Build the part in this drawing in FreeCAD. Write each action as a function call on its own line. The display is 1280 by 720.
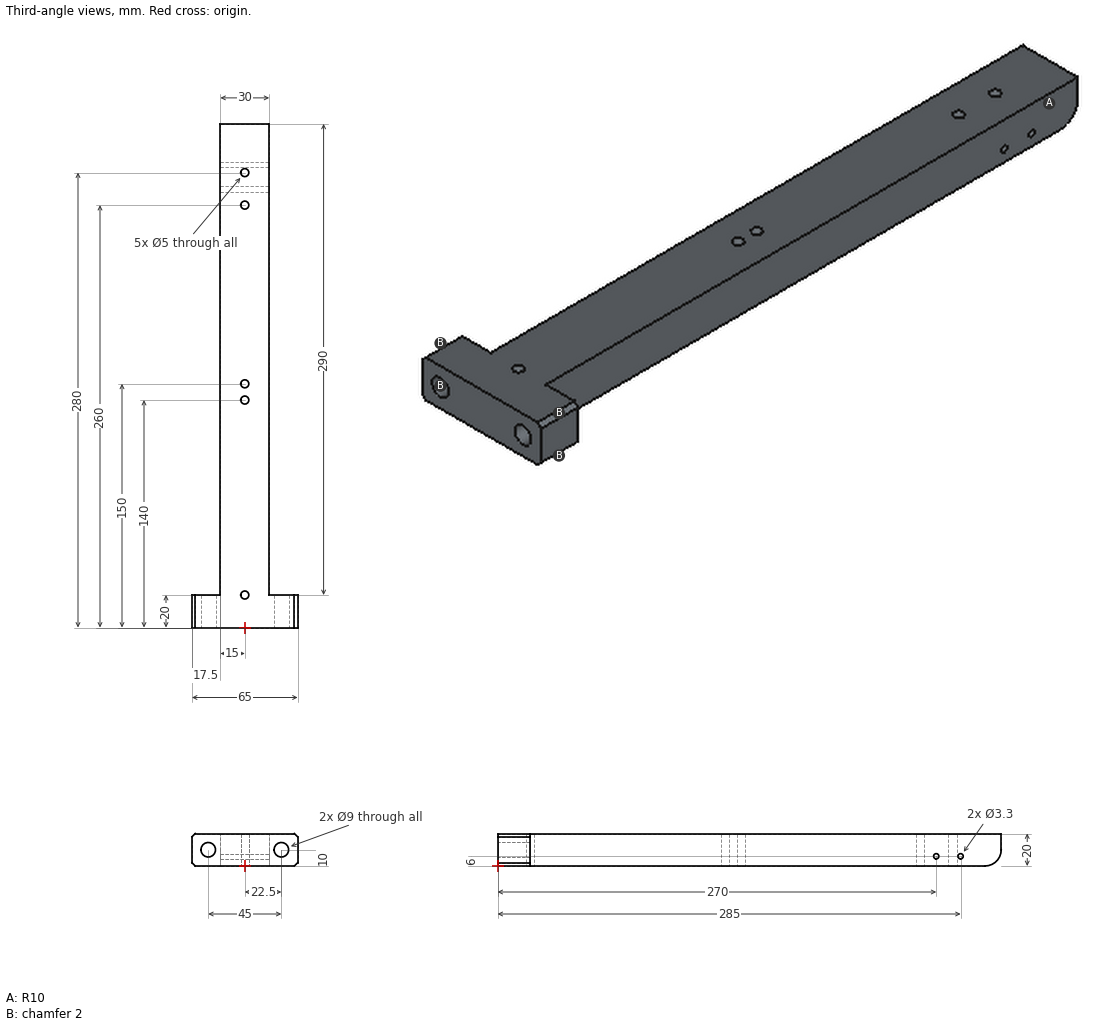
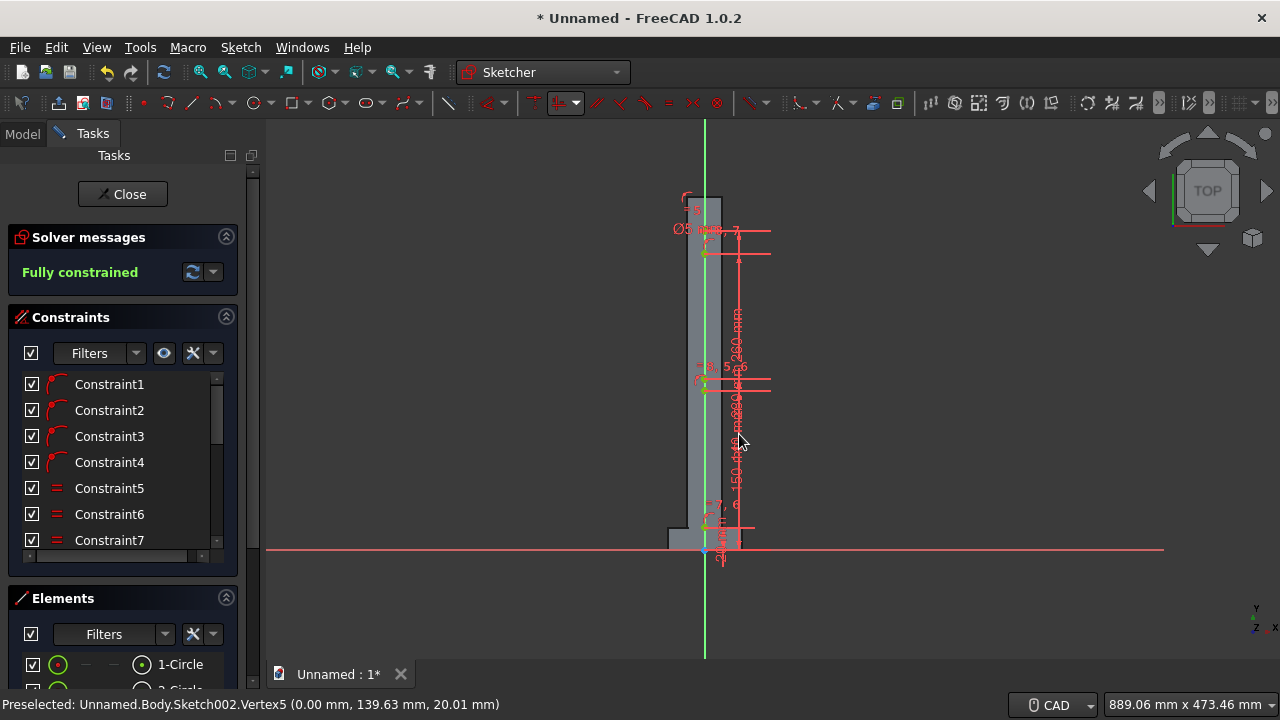
click(123, 194)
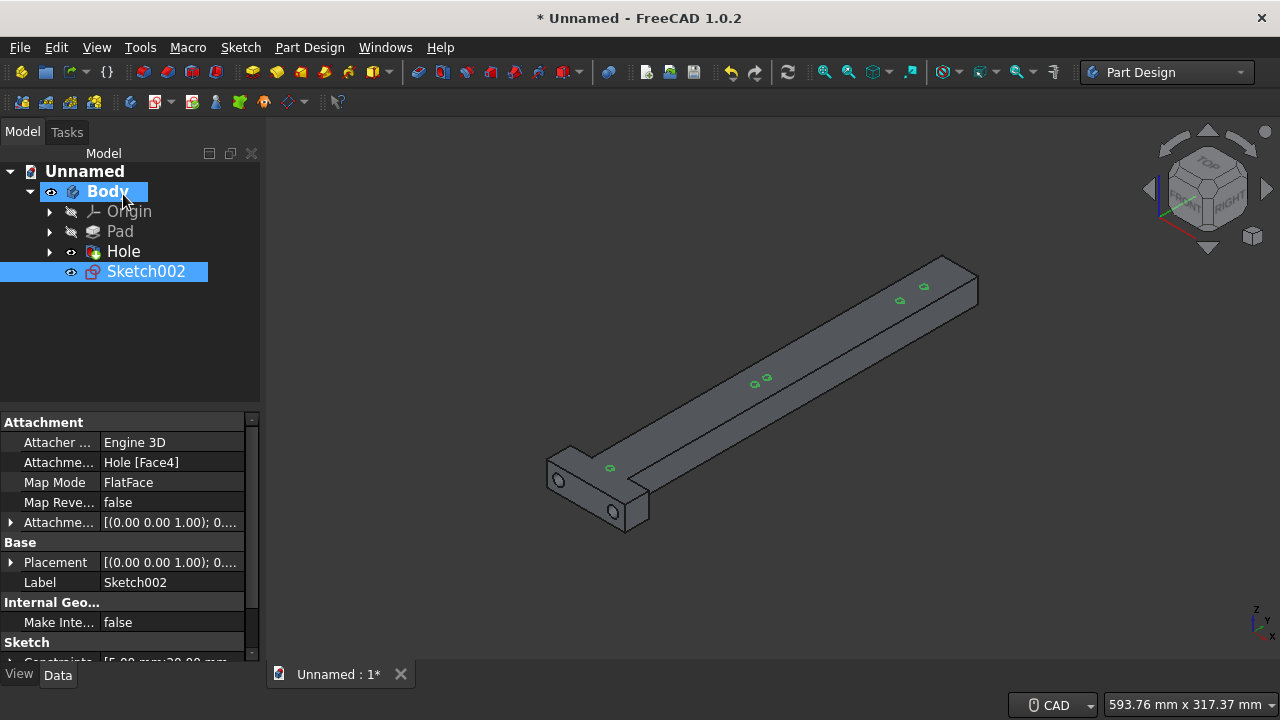
click(444, 72)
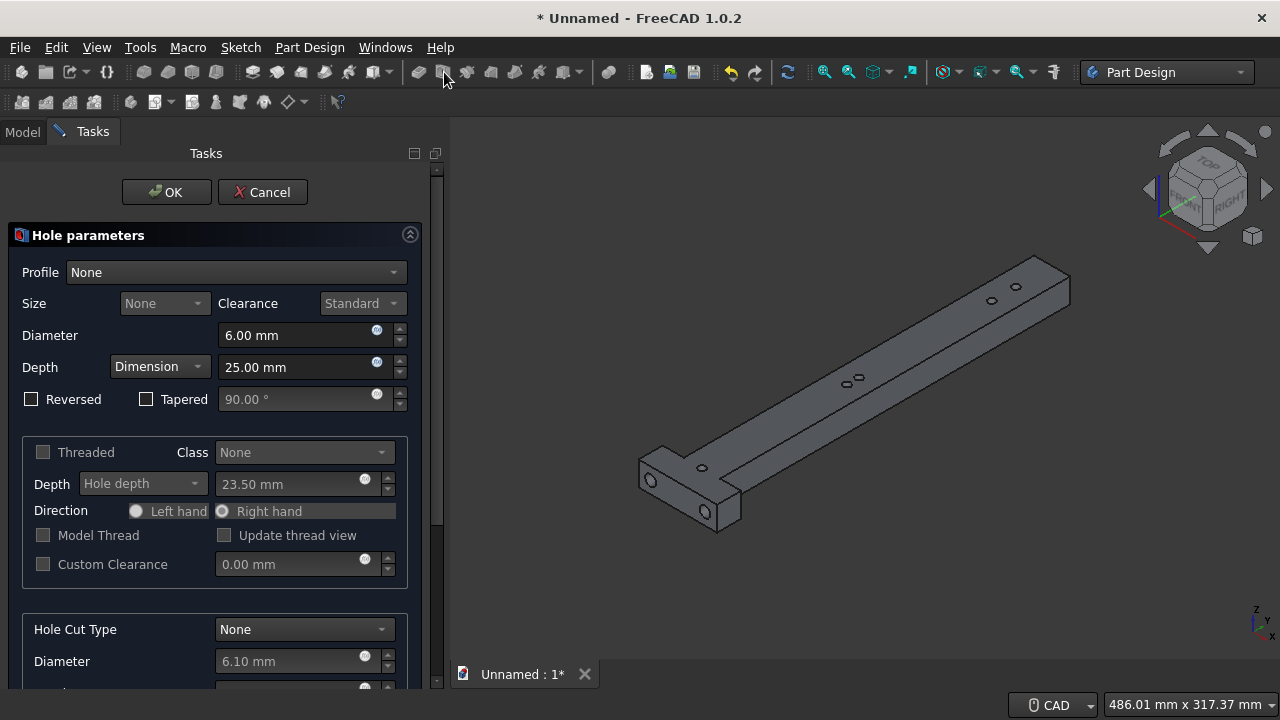
triple_click(305, 335)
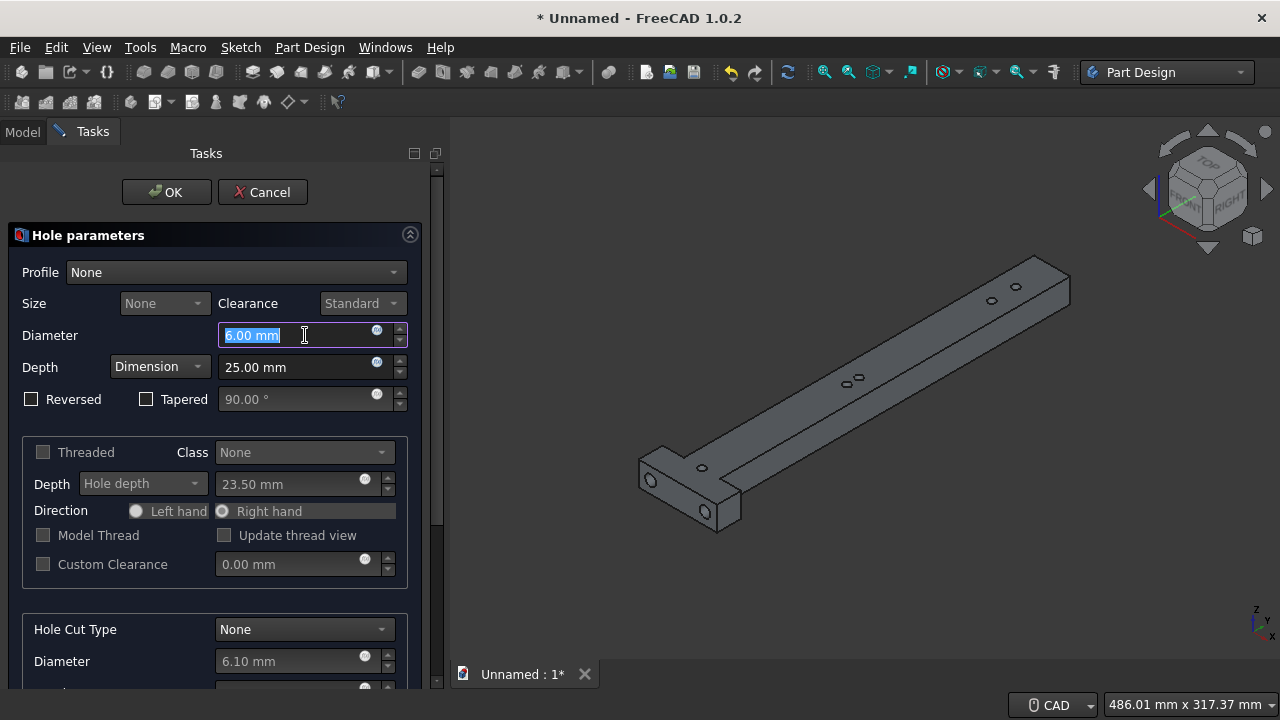
text(5)
key(Tab)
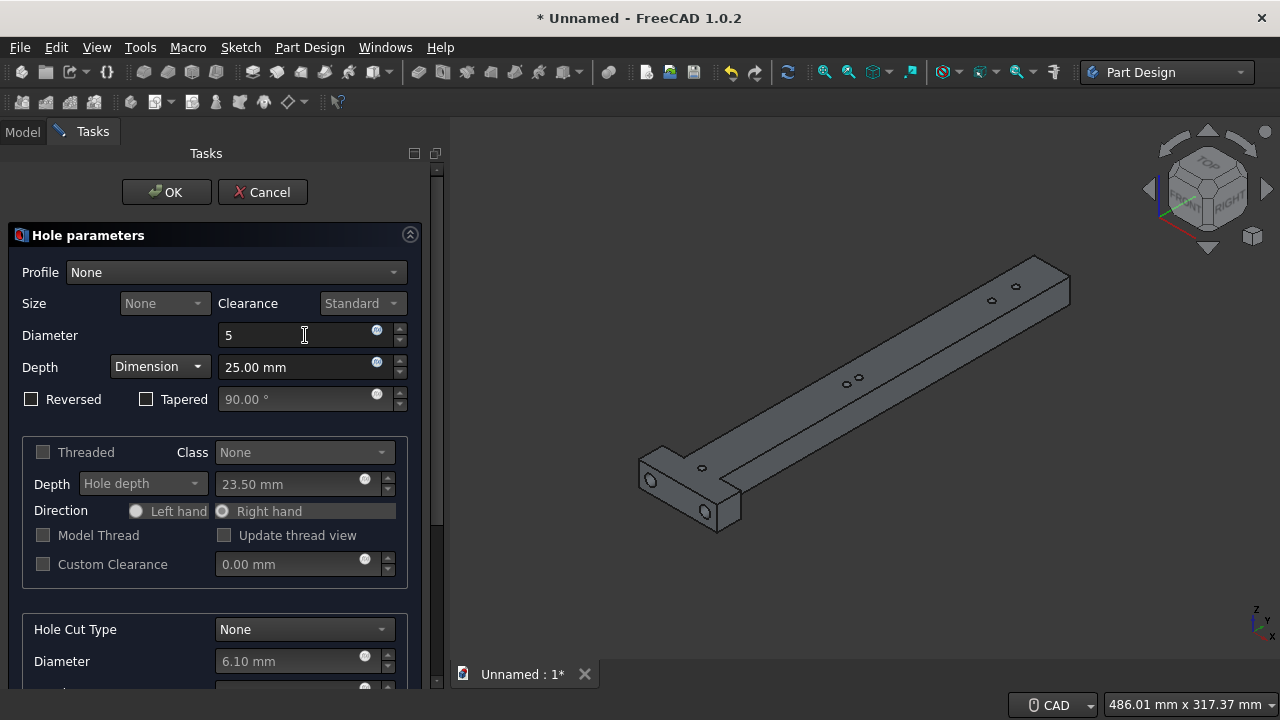
click(161, 366)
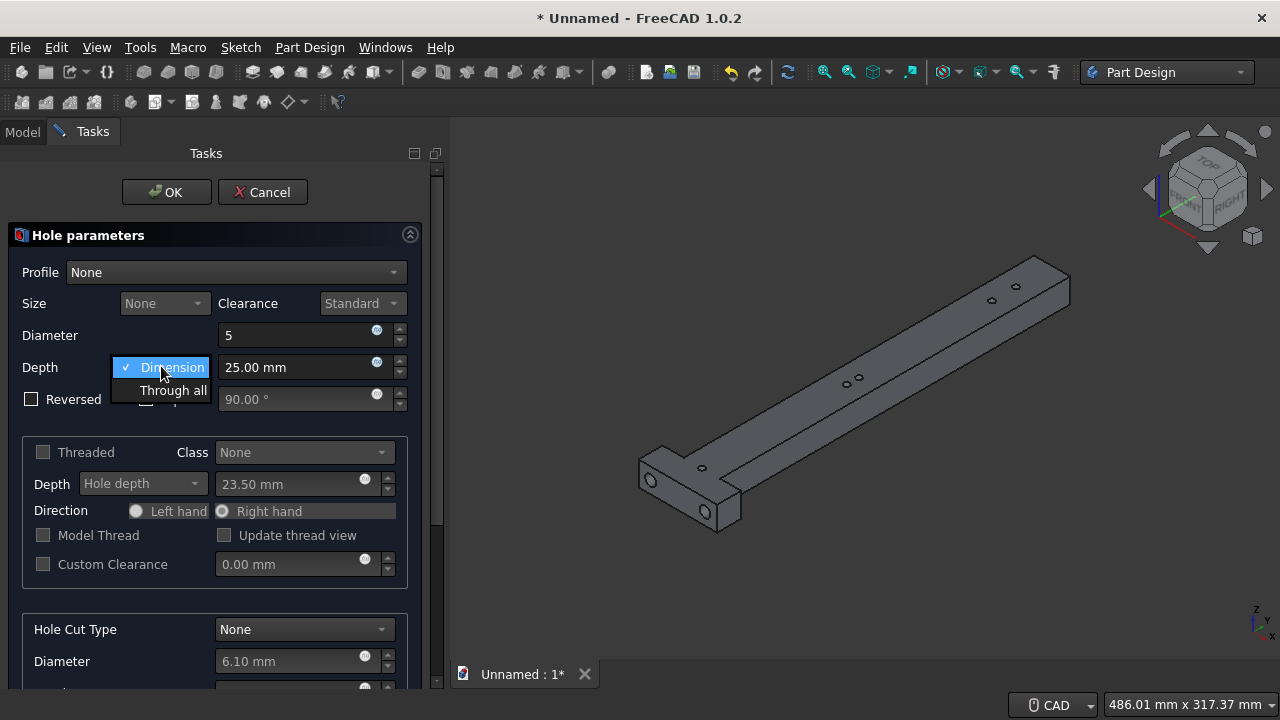
click(160, 390)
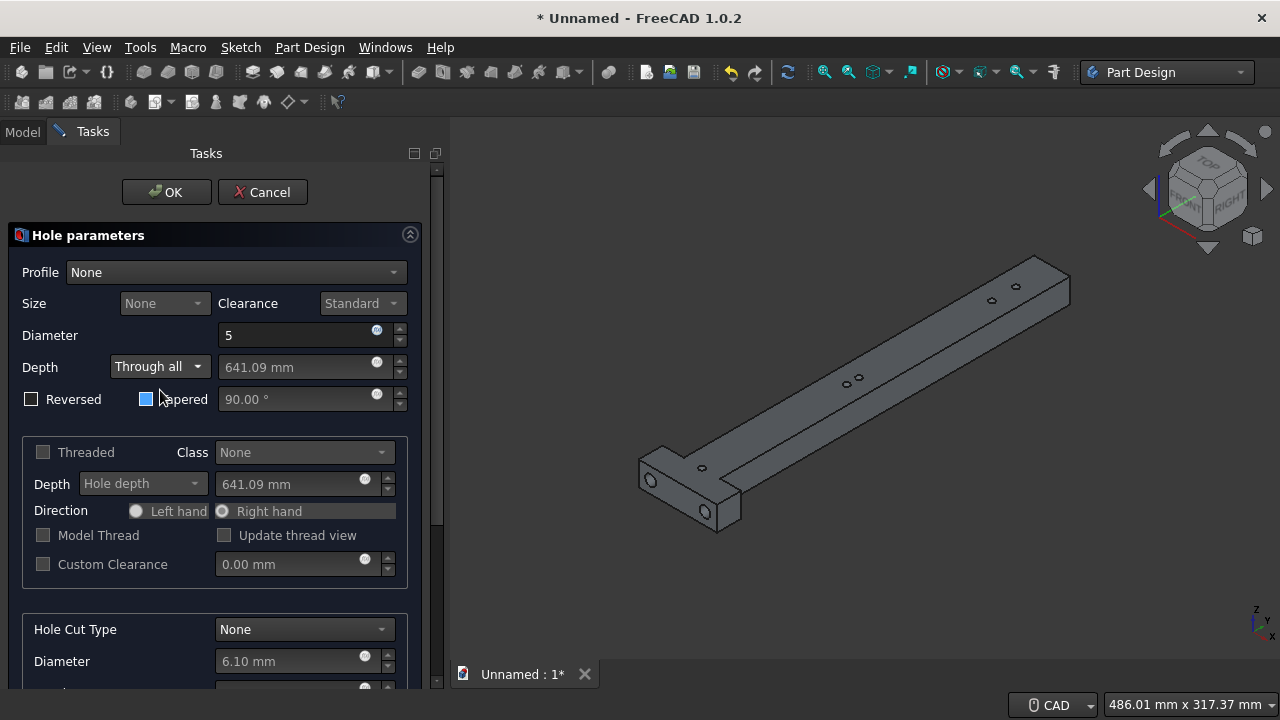
click(167, 192)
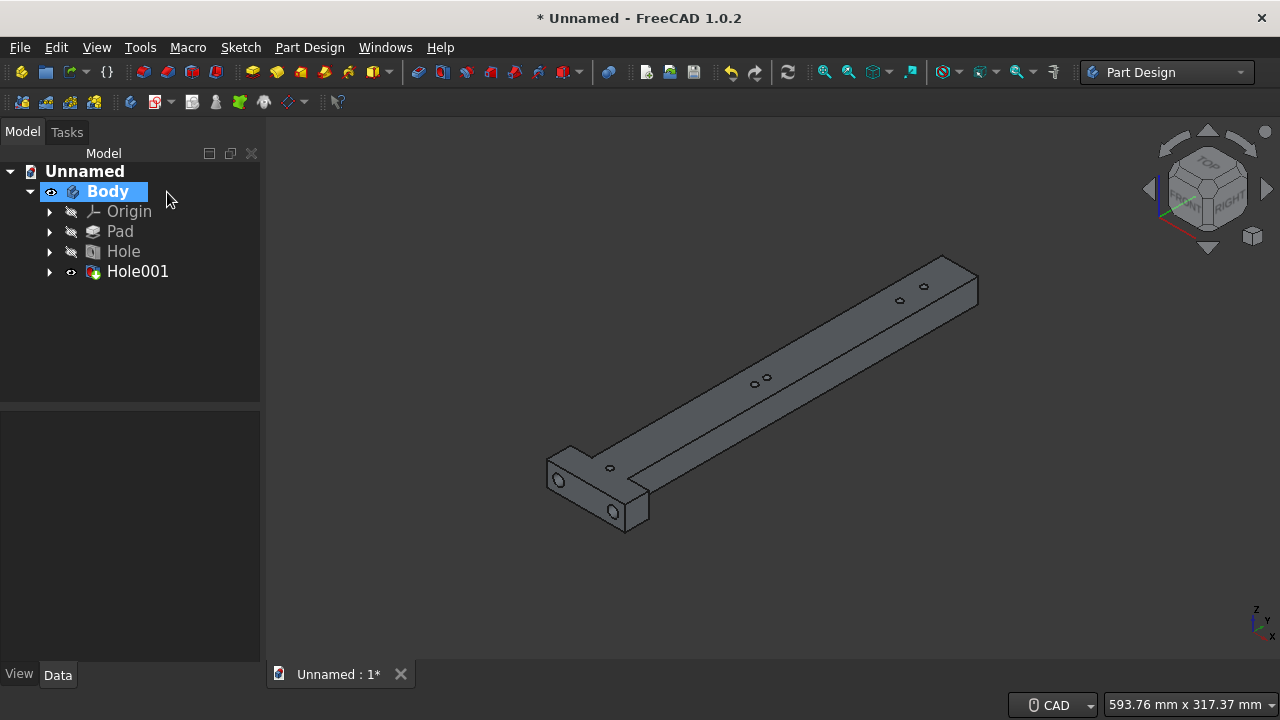
key(2)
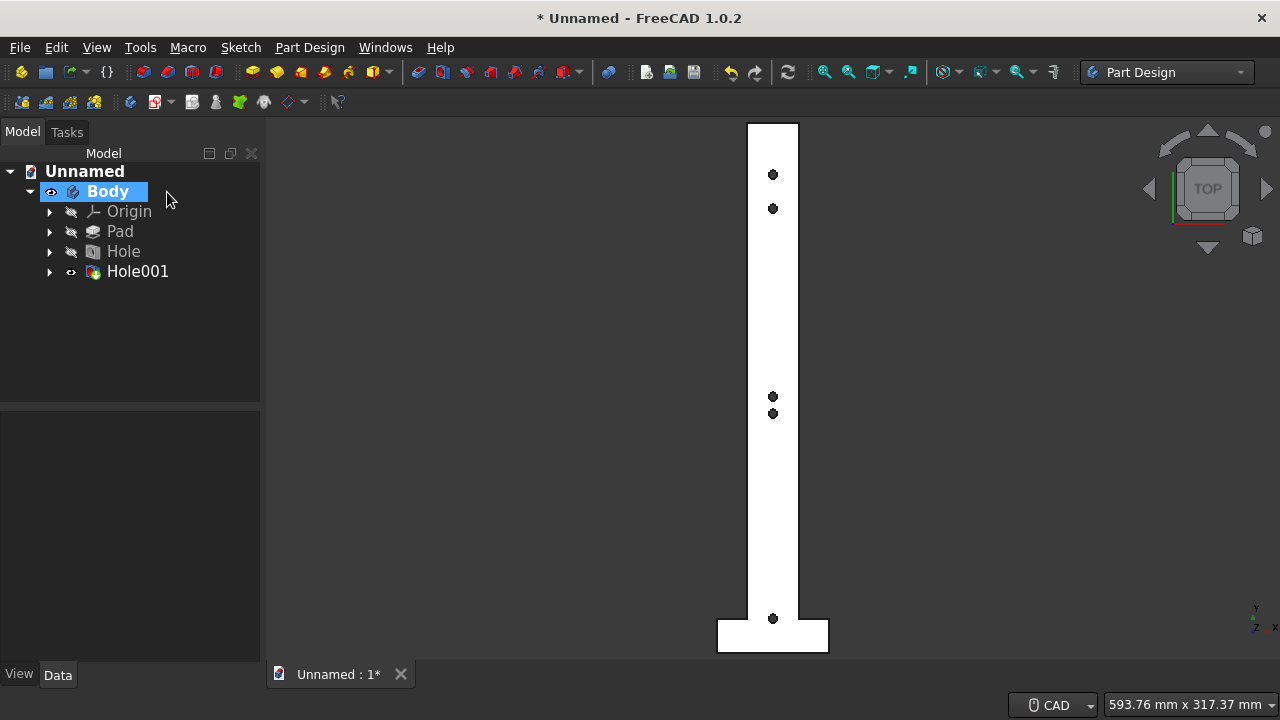
key(0)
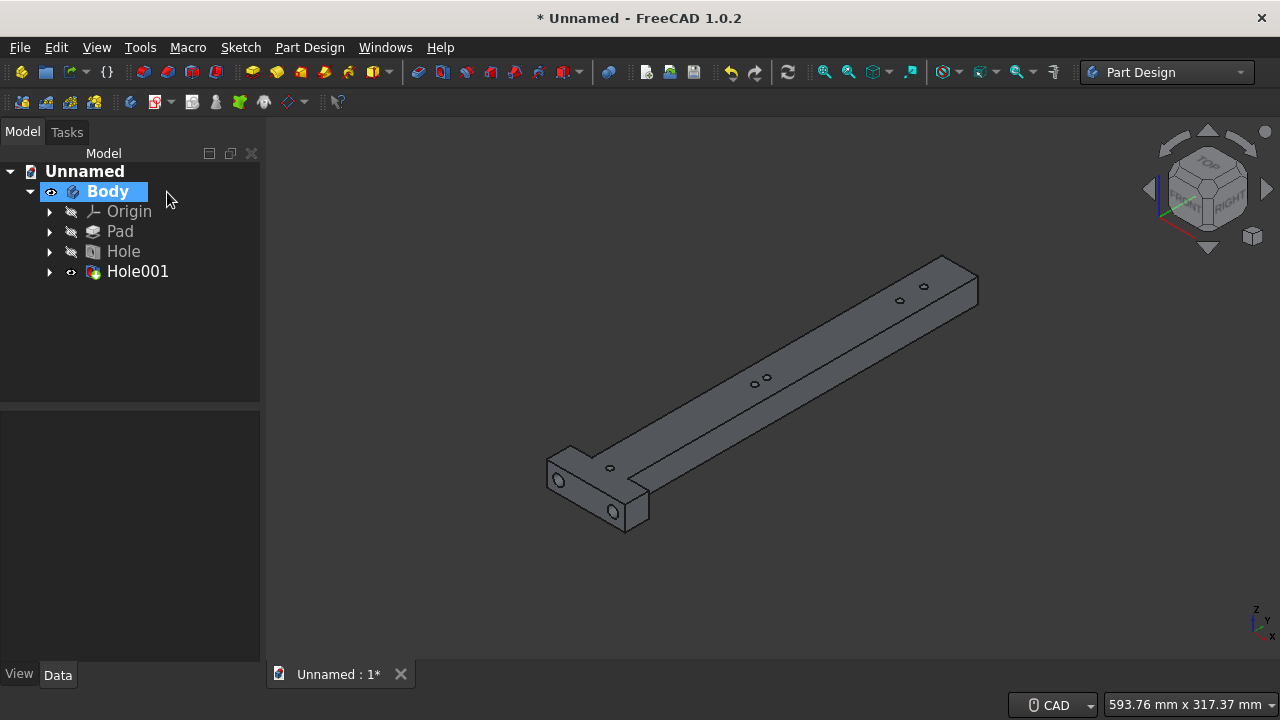
key(1)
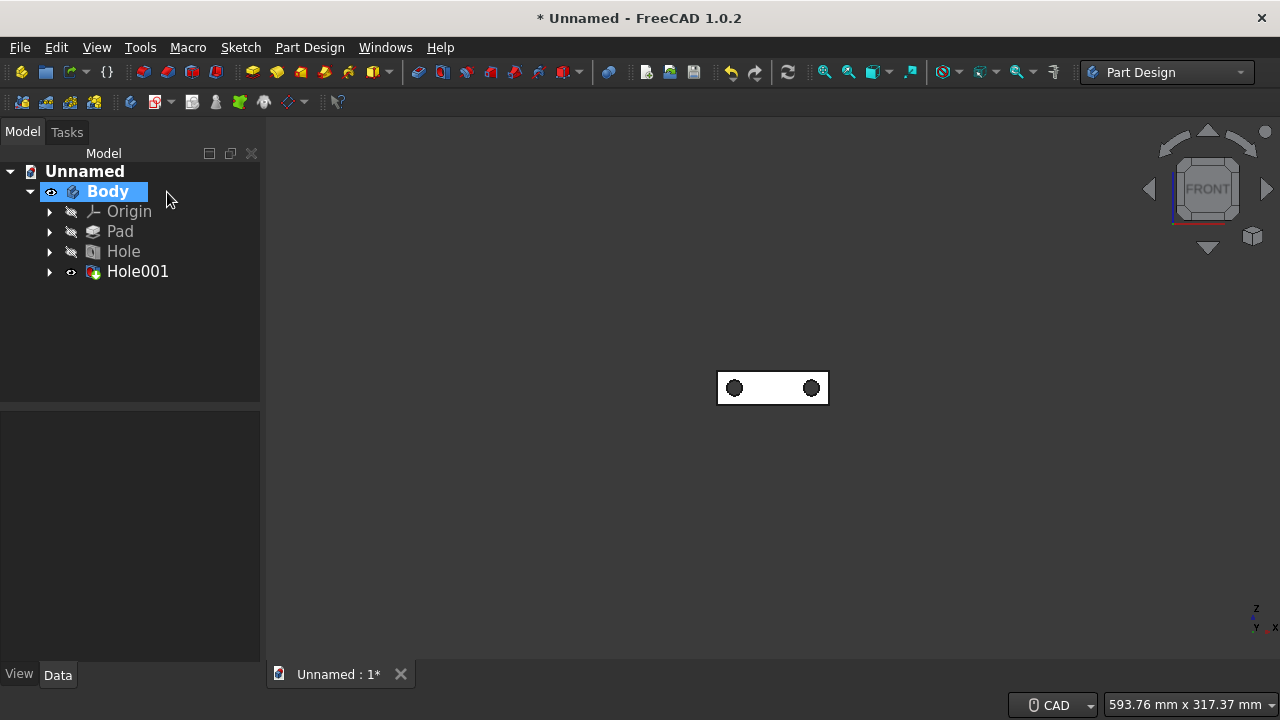
click(826, 72)